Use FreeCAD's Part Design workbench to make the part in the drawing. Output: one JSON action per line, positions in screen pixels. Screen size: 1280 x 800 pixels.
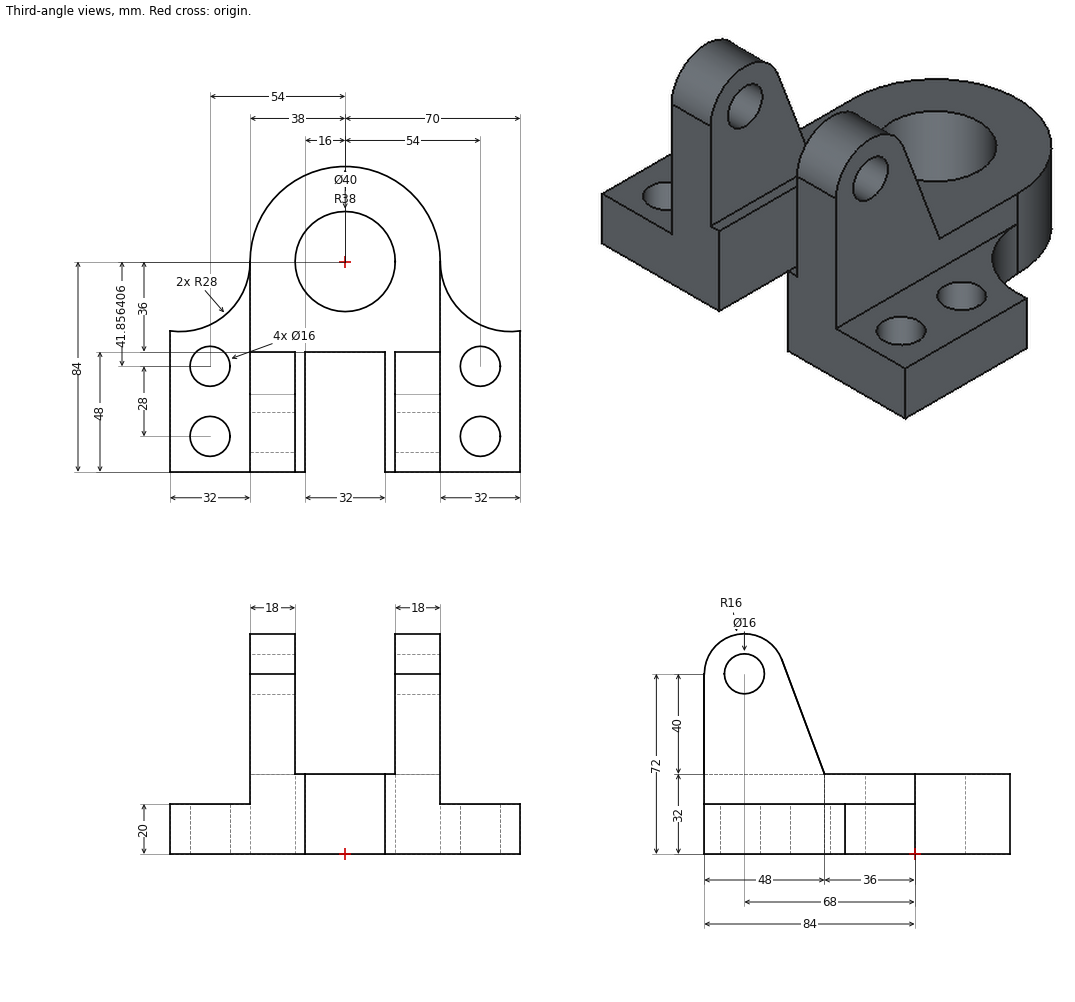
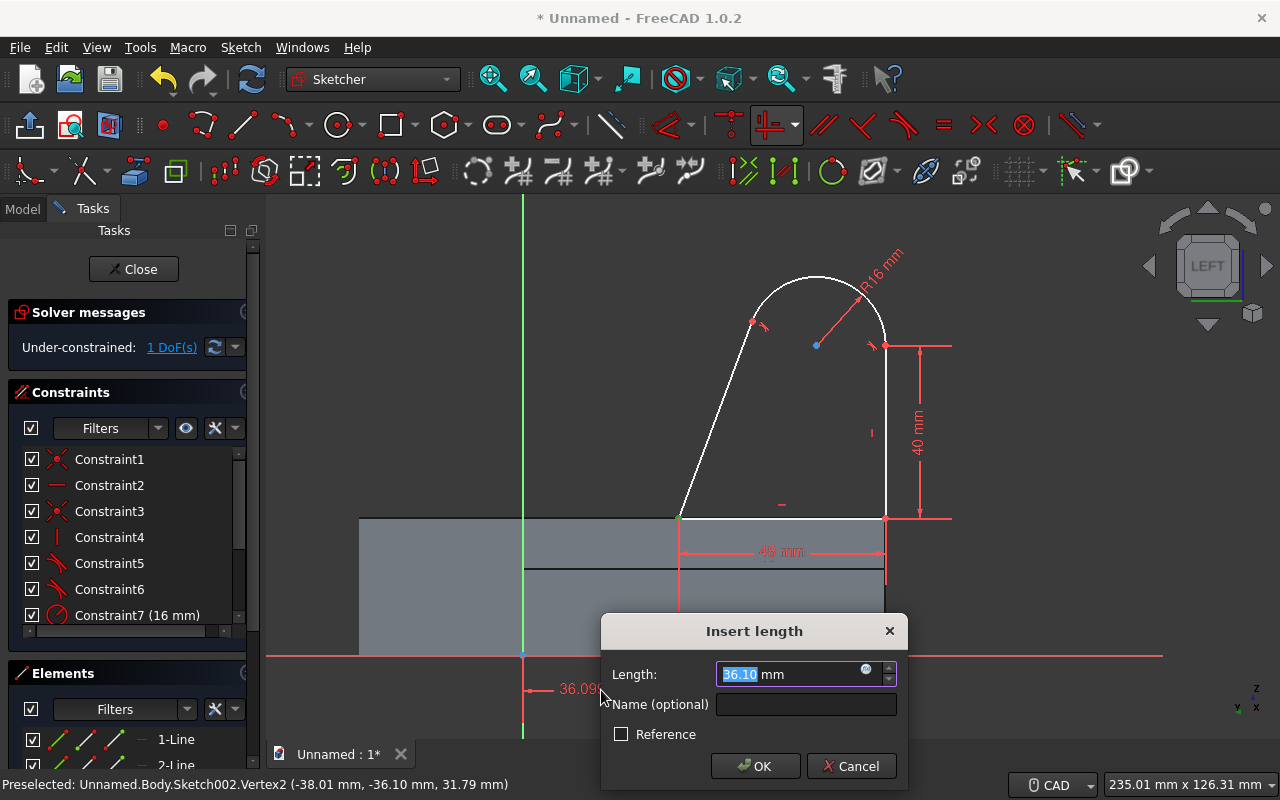
{"action": "type", "text": "36"}
{"action": "key", "text": "Return"}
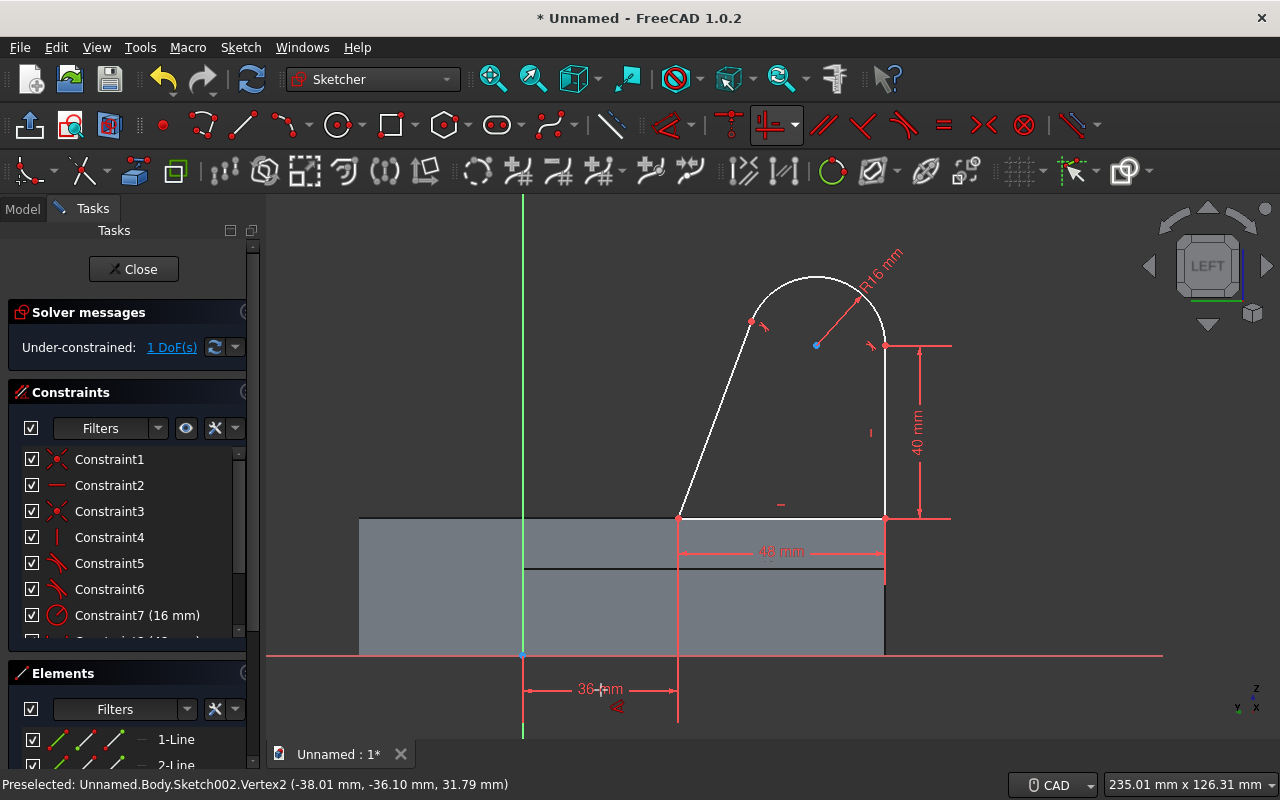
{"action": "left_click", "coordinate": [678, 519]}
{"action": "left_click", "coordinate": [489, 587]}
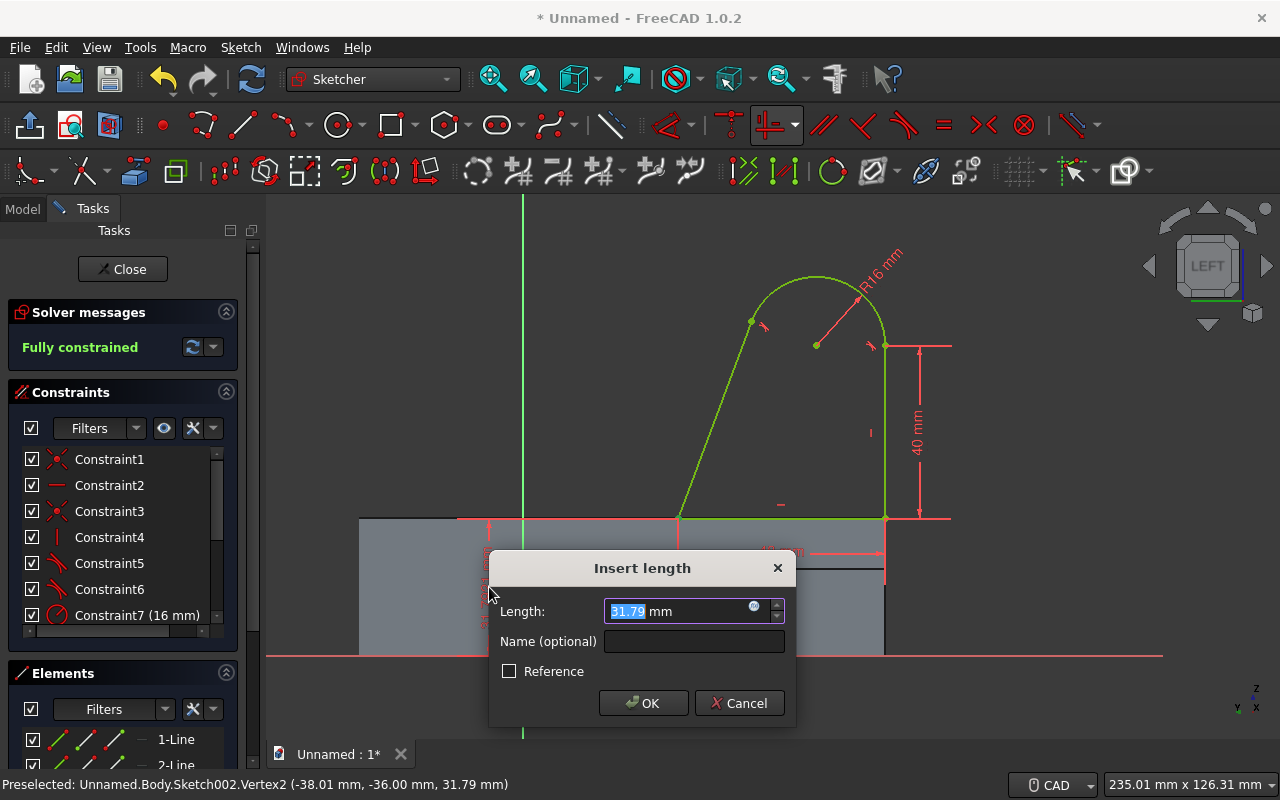
{"action": "type", "text": "32"}
{"action": "key", "text": "Return"}
{"action": "key", "text": "Escape"}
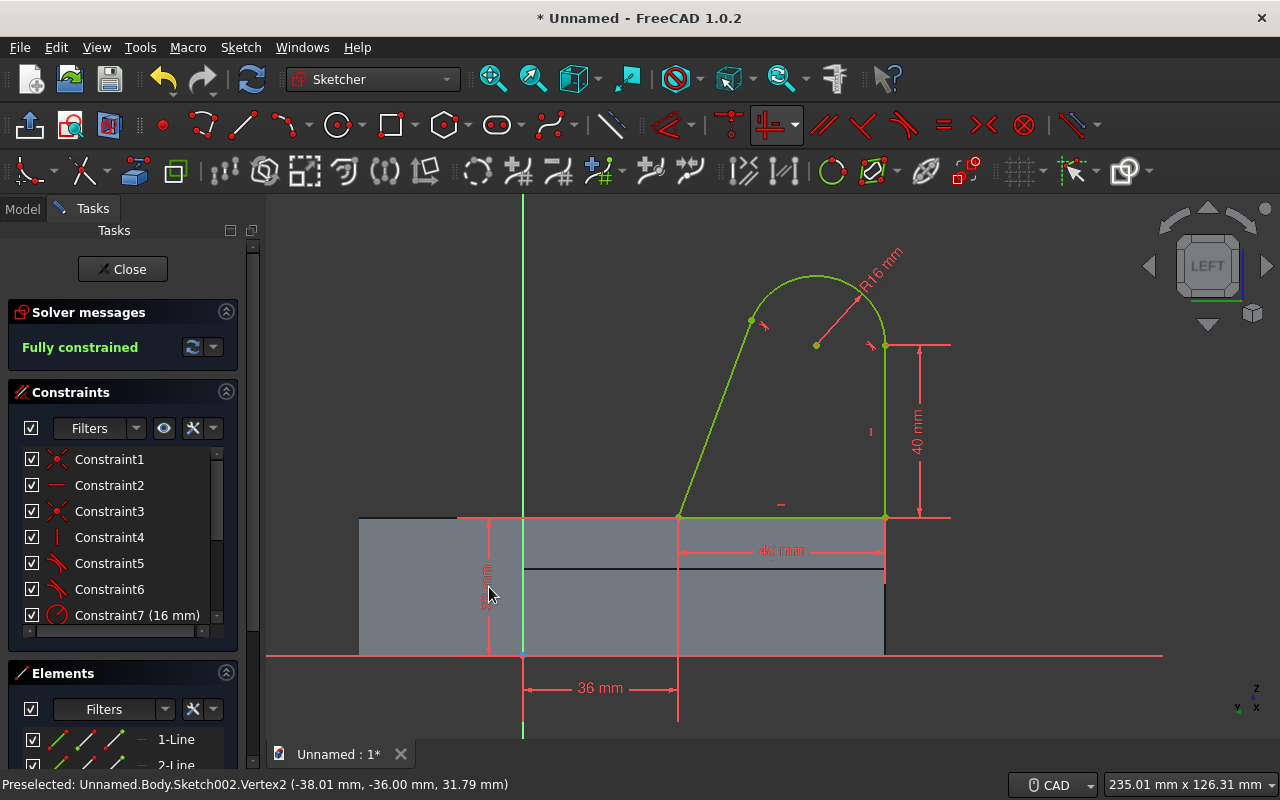
{"action": "left_click", "coordinate": [123, 269]}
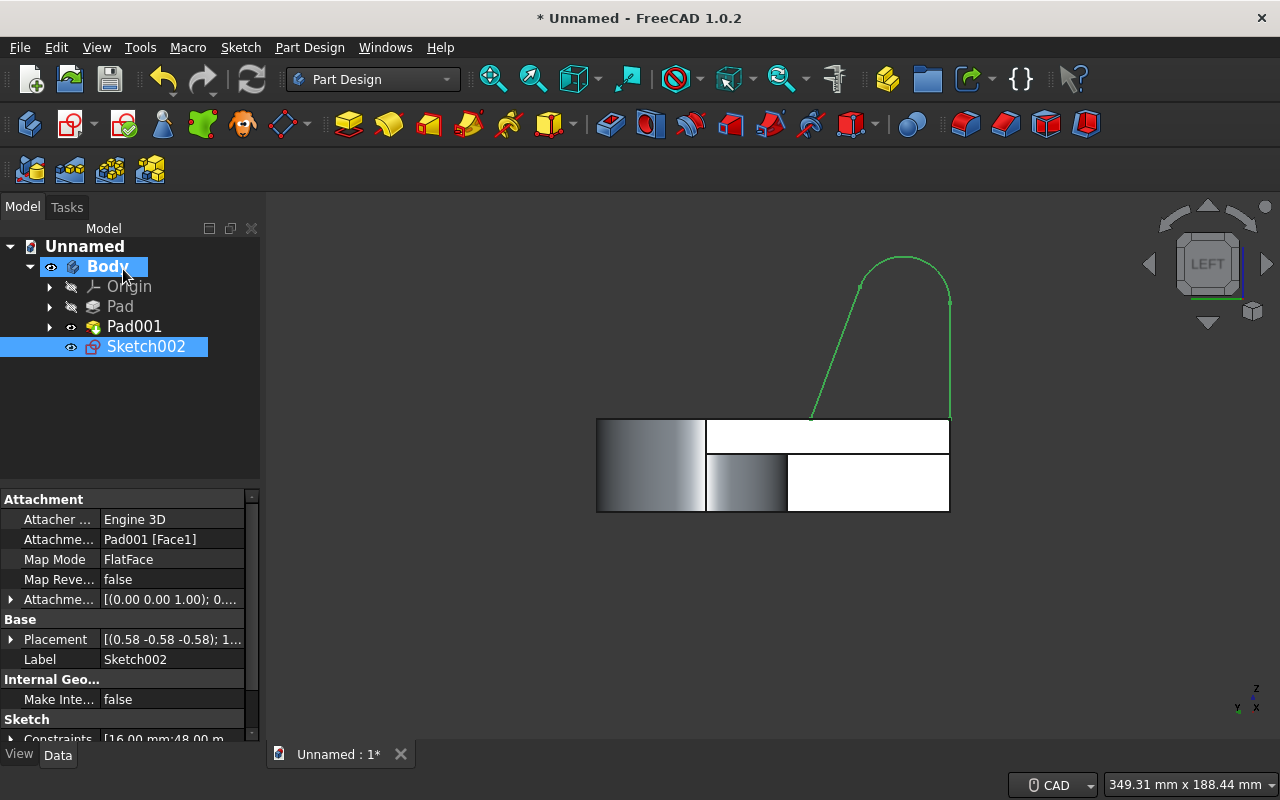
{"action": "left_click", "coordinate": [350, 124]}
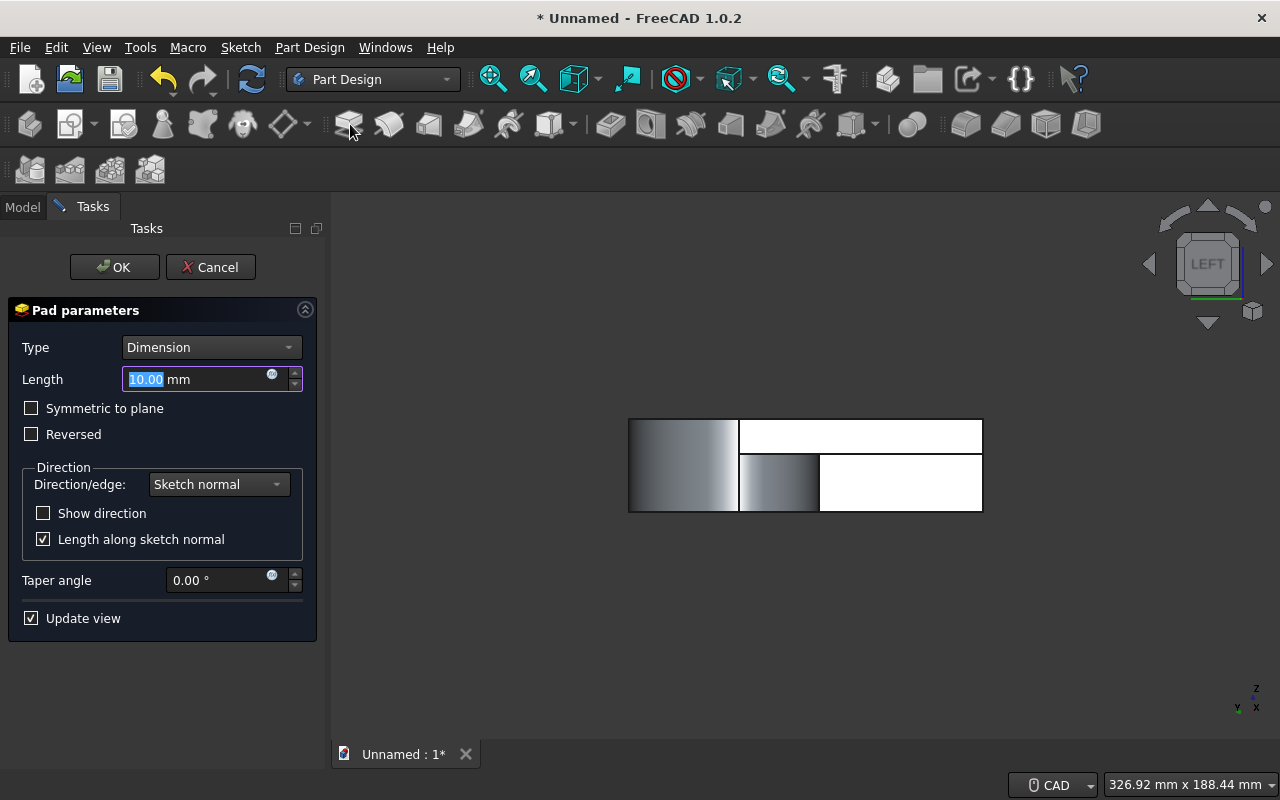
{"action": "type", "text": "18"}
{"action": "key", "text": "Tab"}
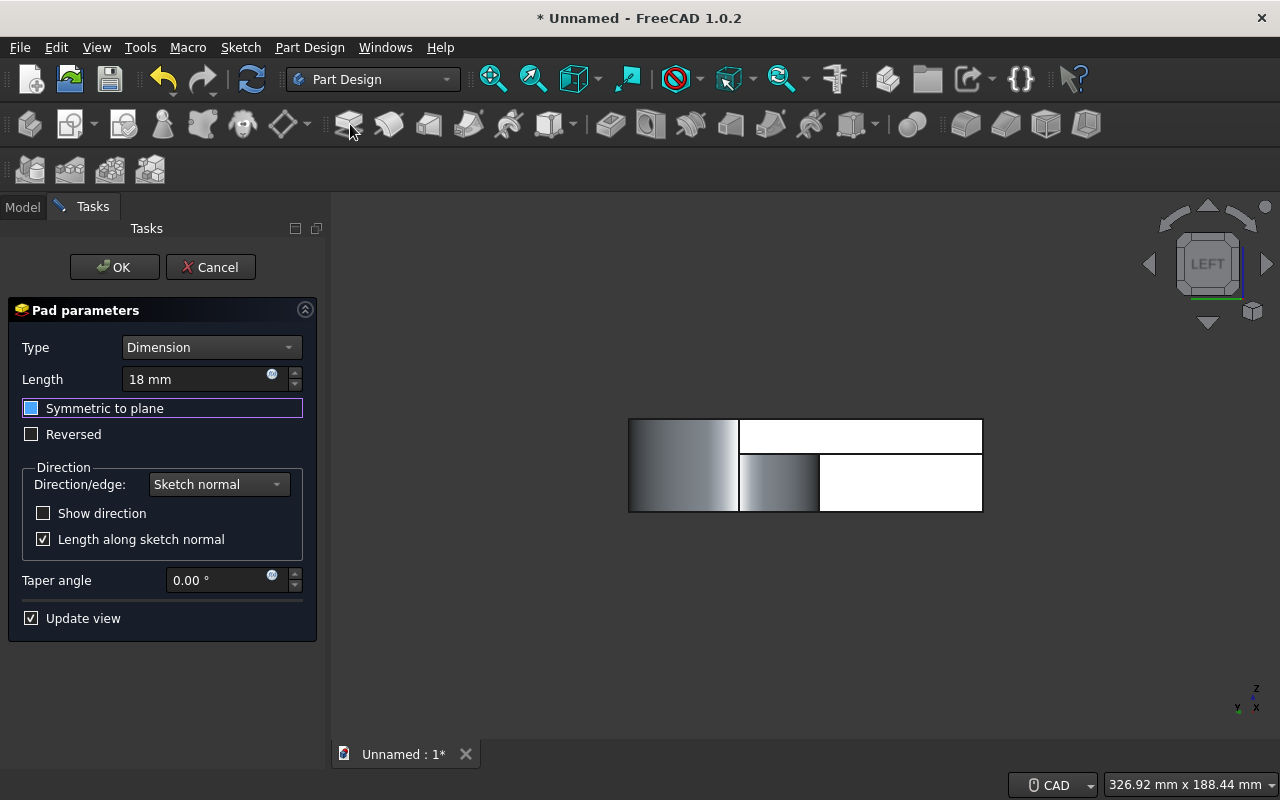
{"action": "left_click", "coordinate": [30, 434]}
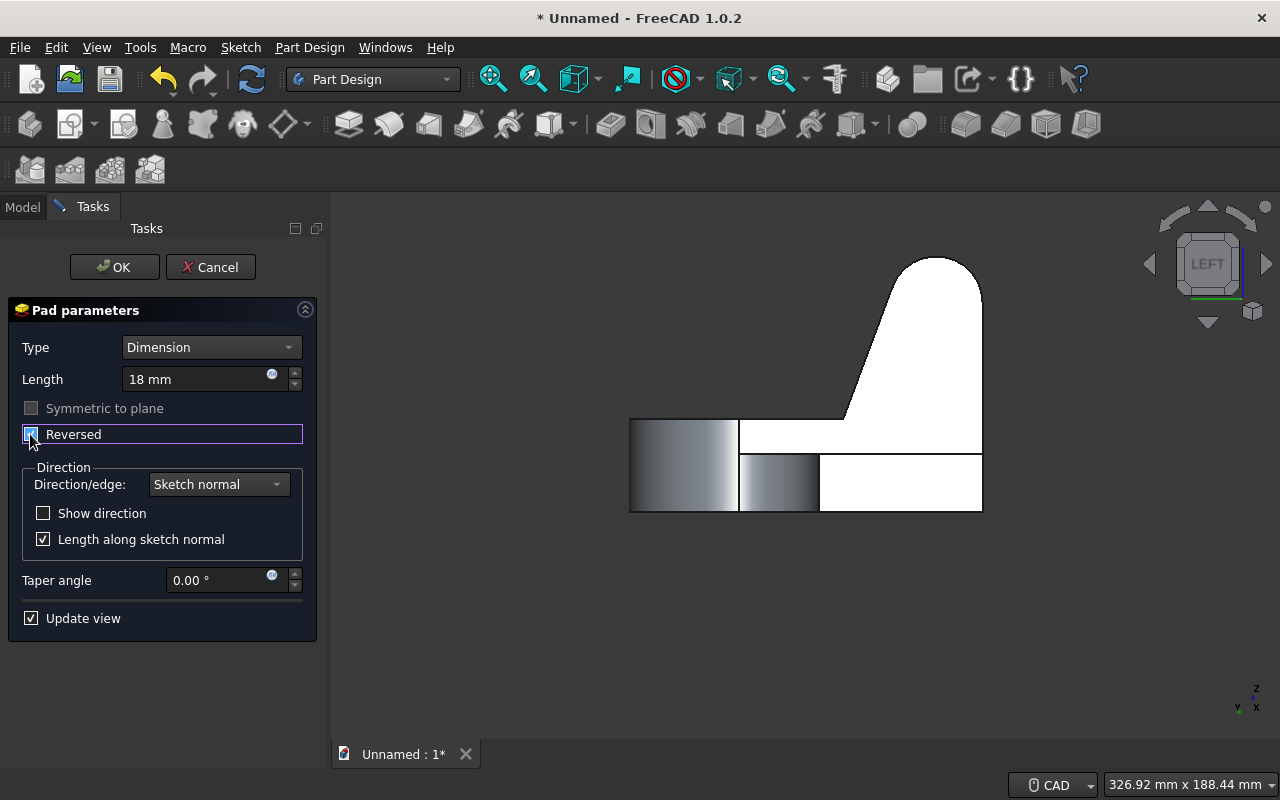
{"action": "left_click", "coordinate": [115, 267]}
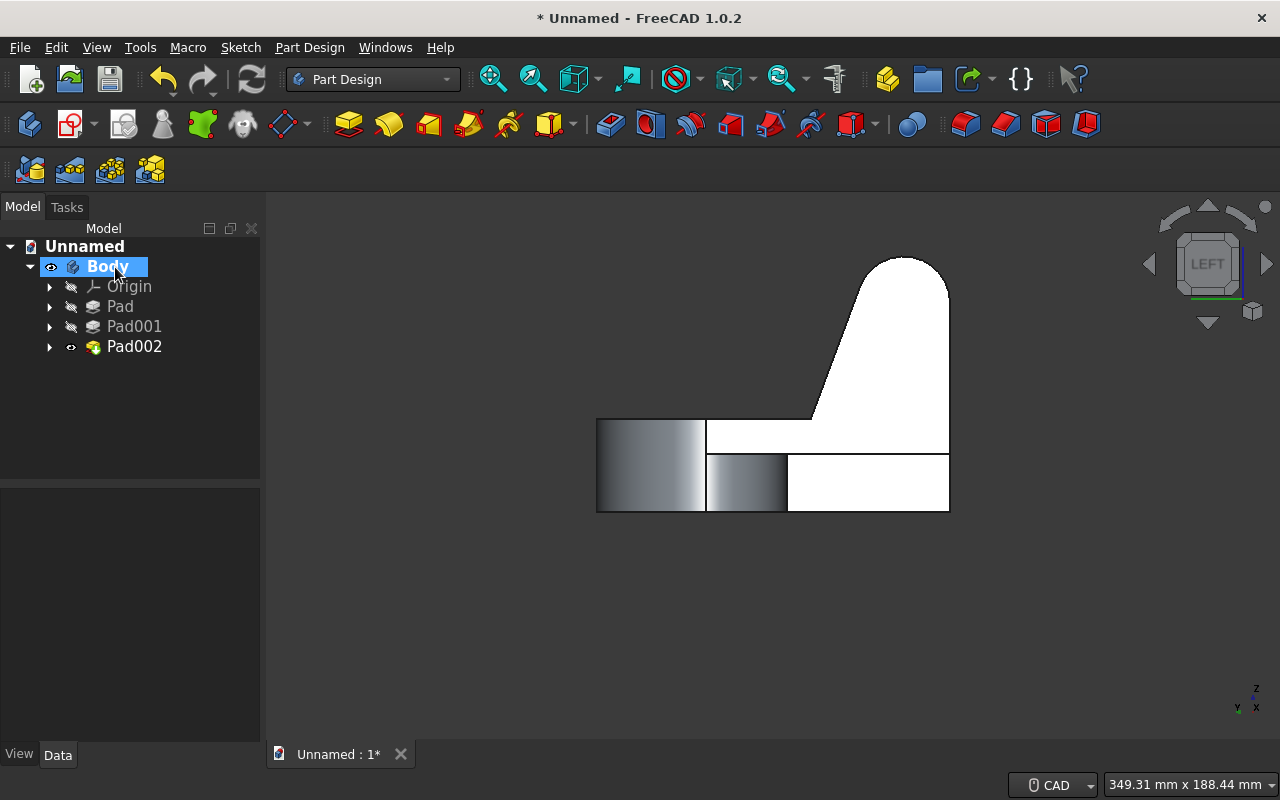
{"action": "left_click", "coordinate": [50, 287]}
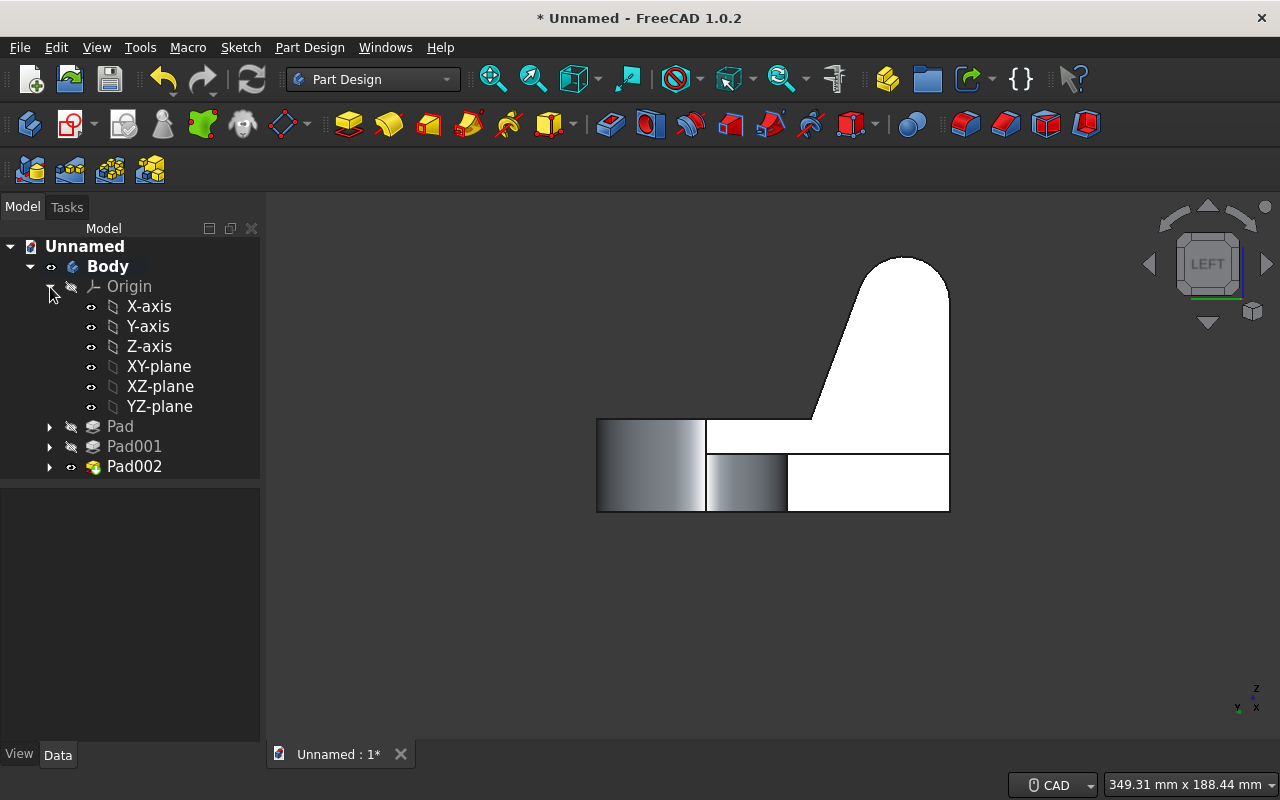
{"action": "left_click", "coordinate": [136, 407]}